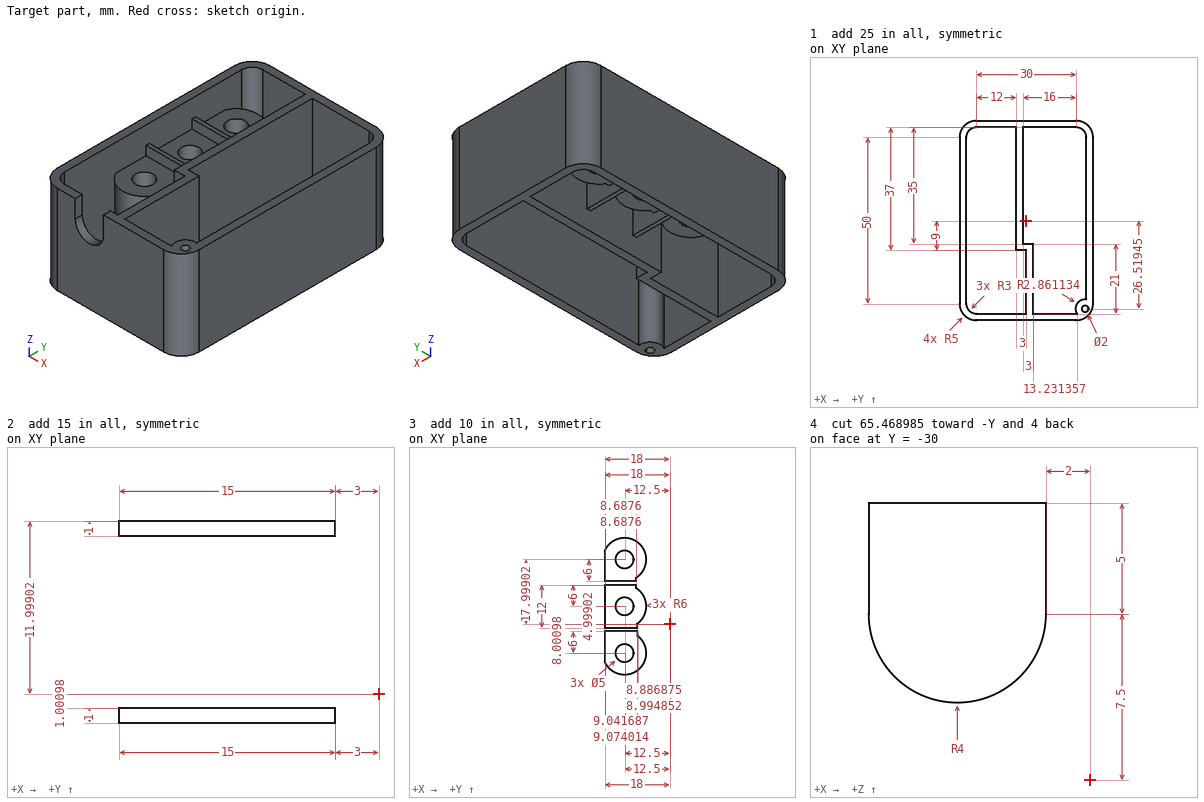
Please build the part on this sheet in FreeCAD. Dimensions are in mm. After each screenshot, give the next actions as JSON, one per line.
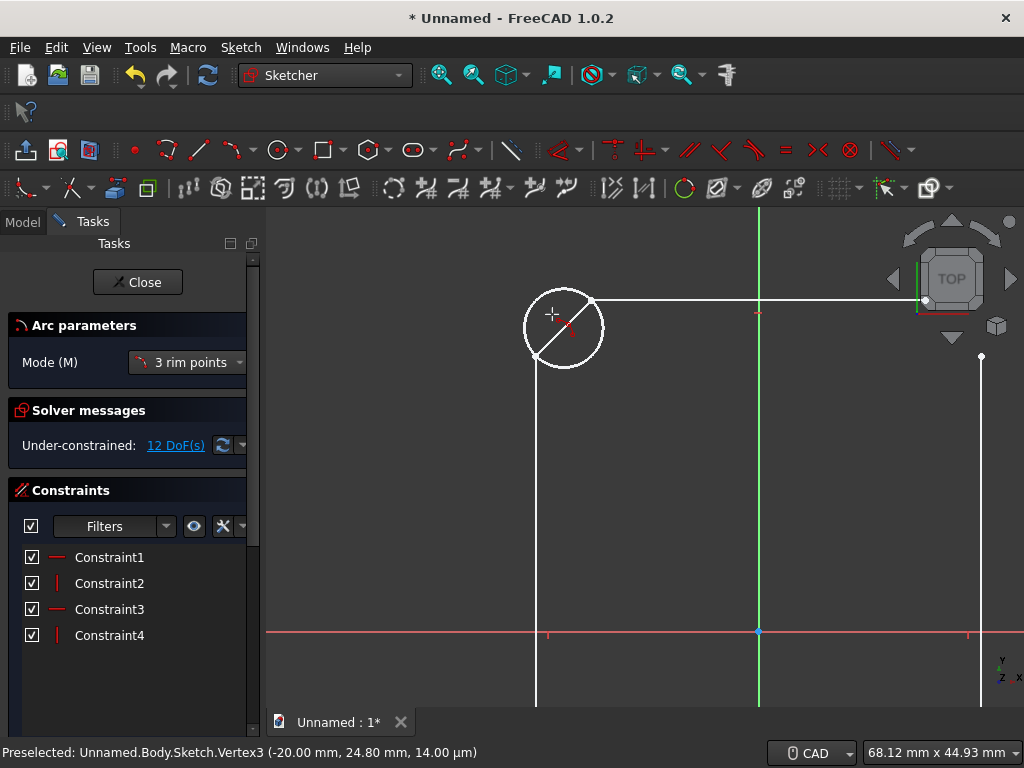
{"action": "left_click", "coordinate": [552, 314]}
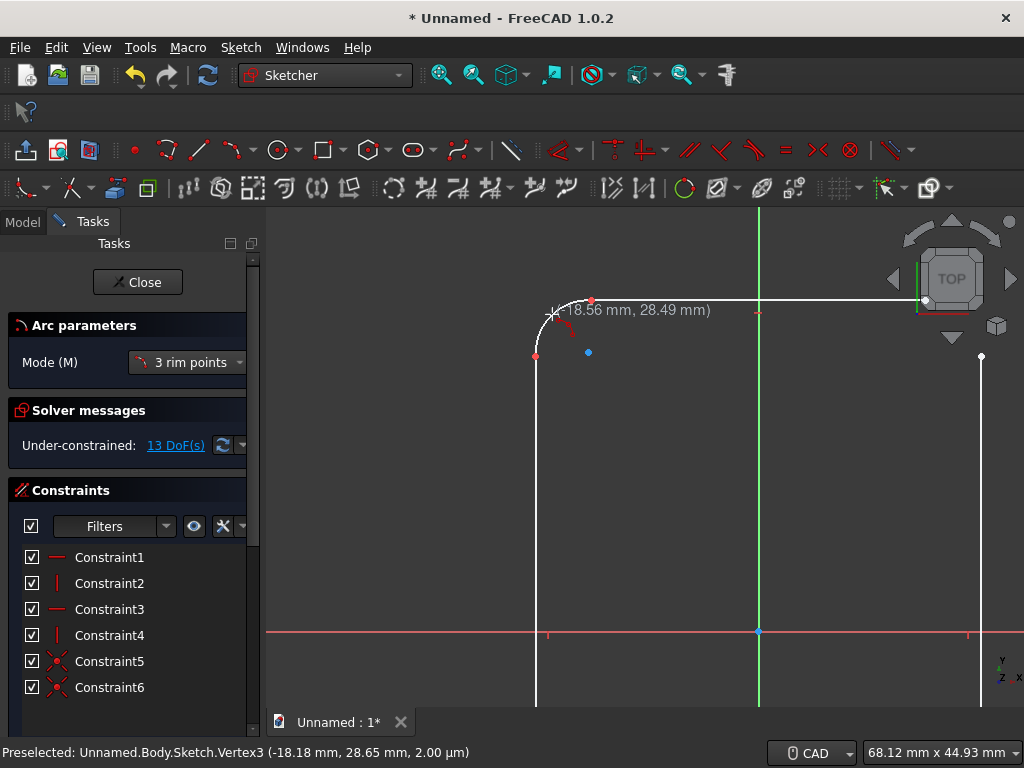
{"action": "scroll", "coordinate": [428, 314], "scroll_direction": "down", "scroll_amount": 4}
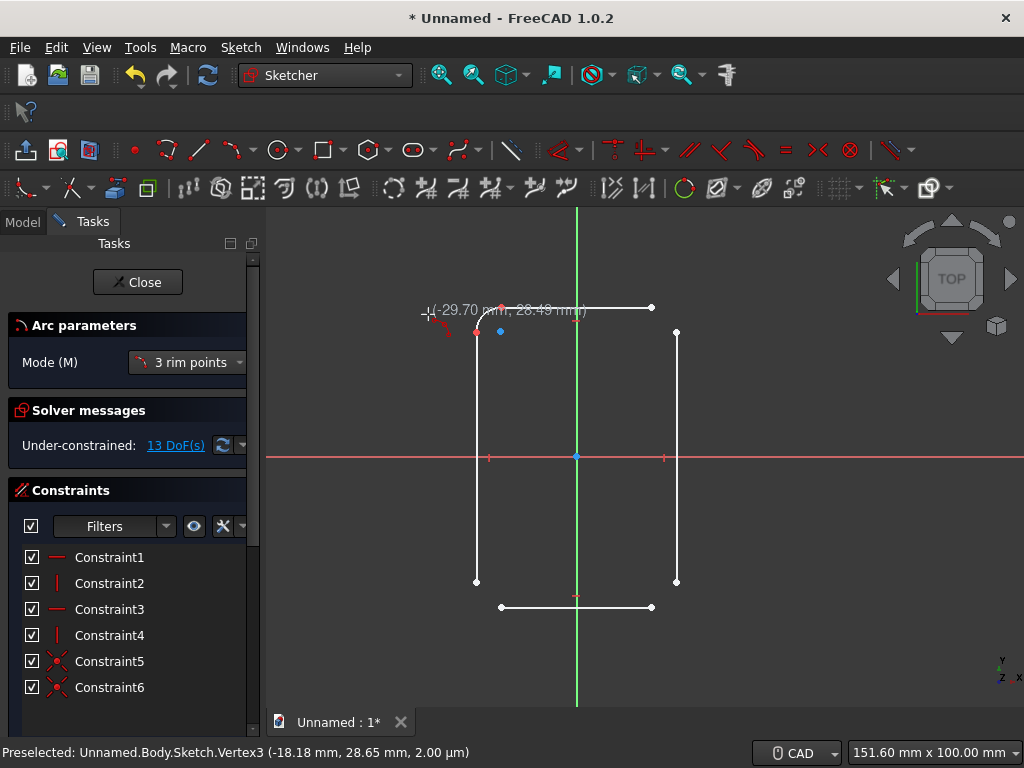
{"action": "left_click", "coordinate": [477, 583]}
{"action": "left_click", "coordinate": [502, 608]}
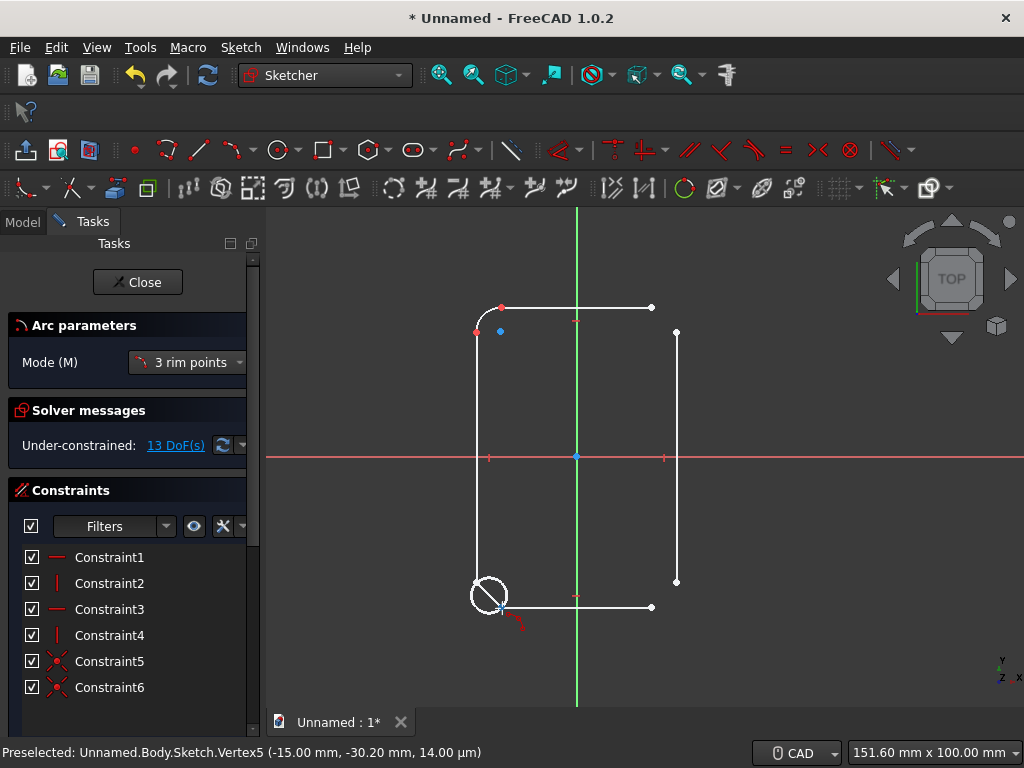
{"action": "scroll", "coordinate": [484, 600], "scroll_direction": "up", "scroll_amount": 4}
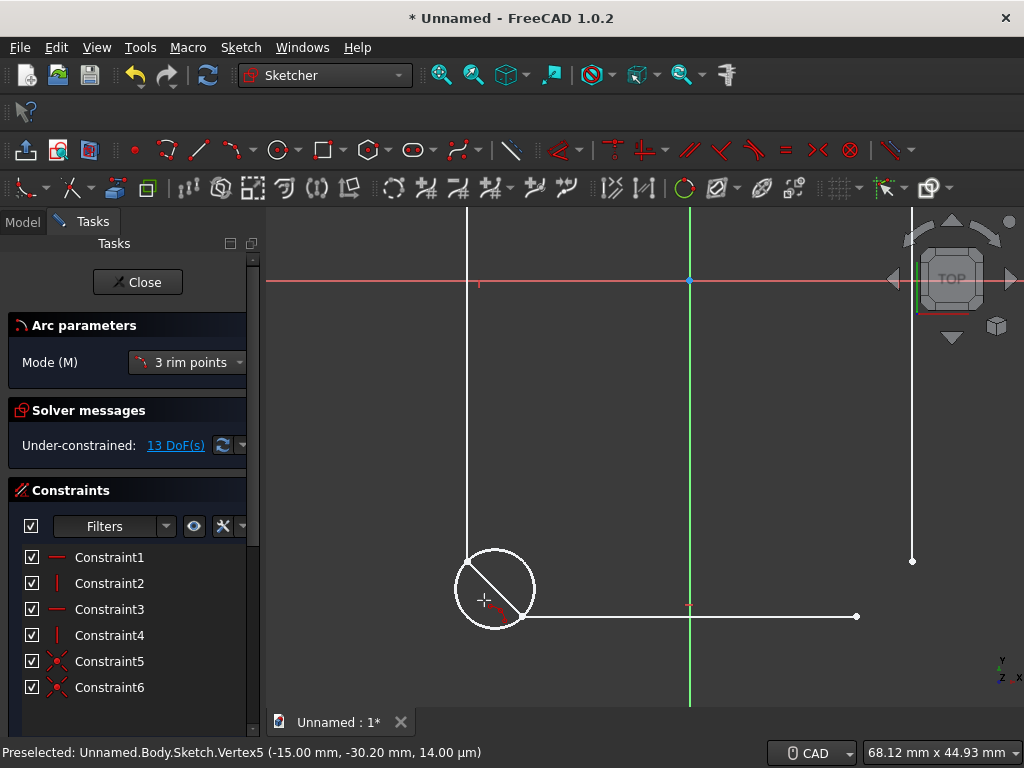
{"action": "left_click", "coordinate": [484, 598]}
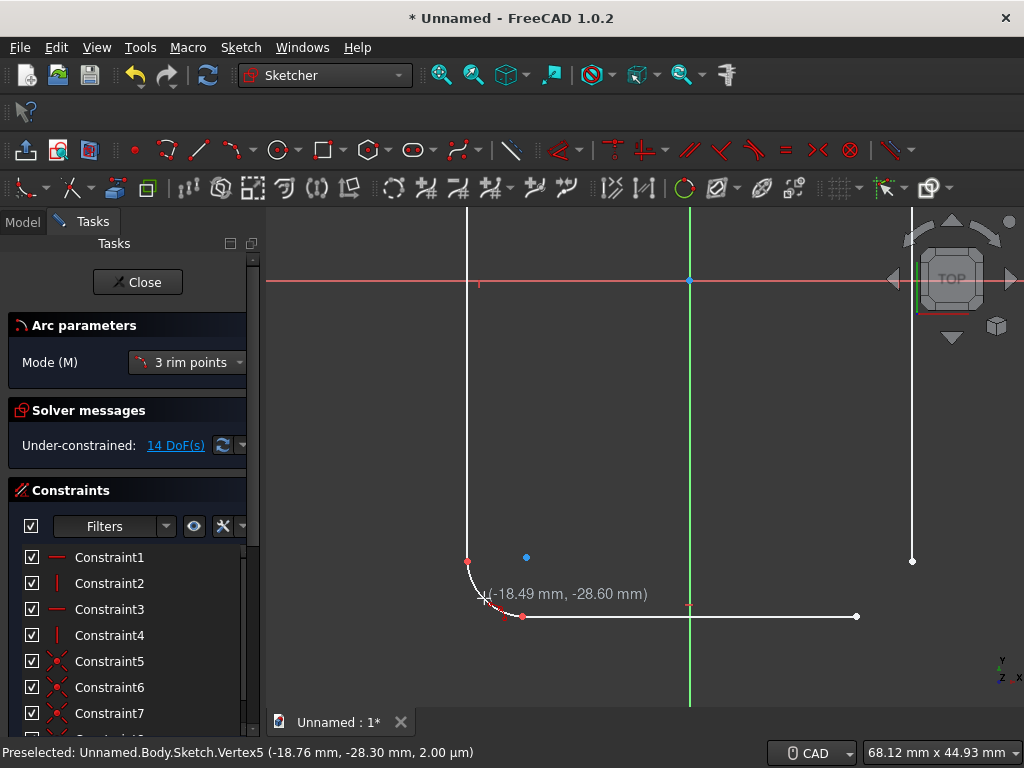
{"action": "left_click", "coordinate": [857, 617]}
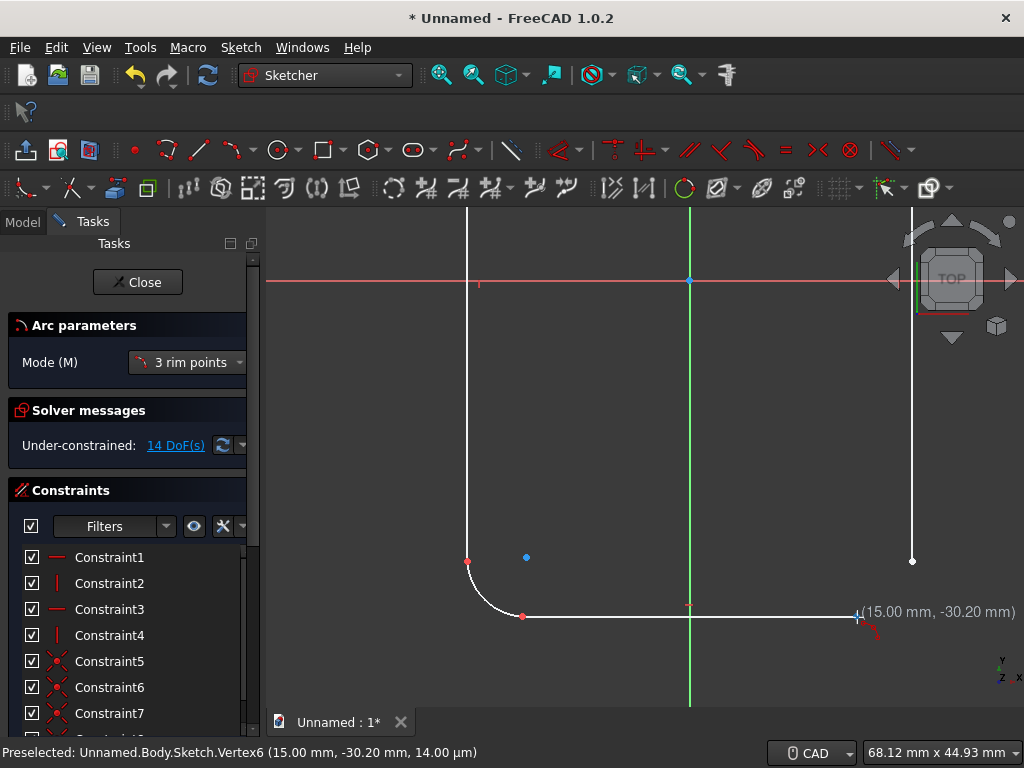
{"action": "scroll", "coordinate": [484, 601], "scroll_direction": "down", "scroll_amount": 4}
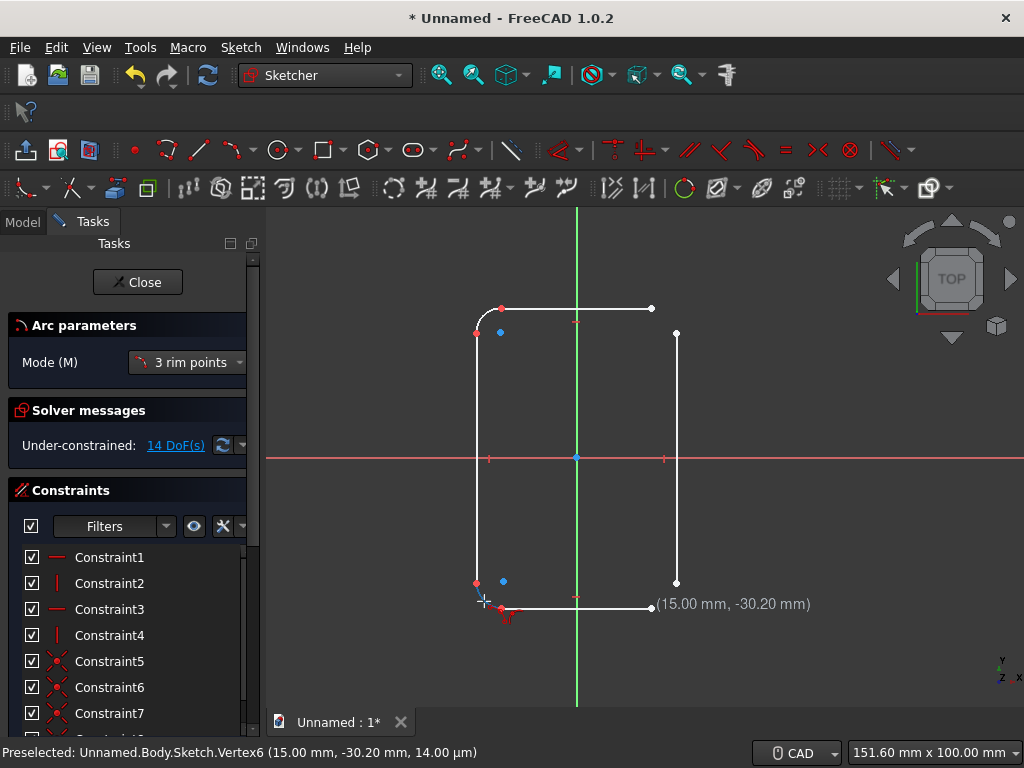
{"action": "left_click", "coordinate": [677, 584]}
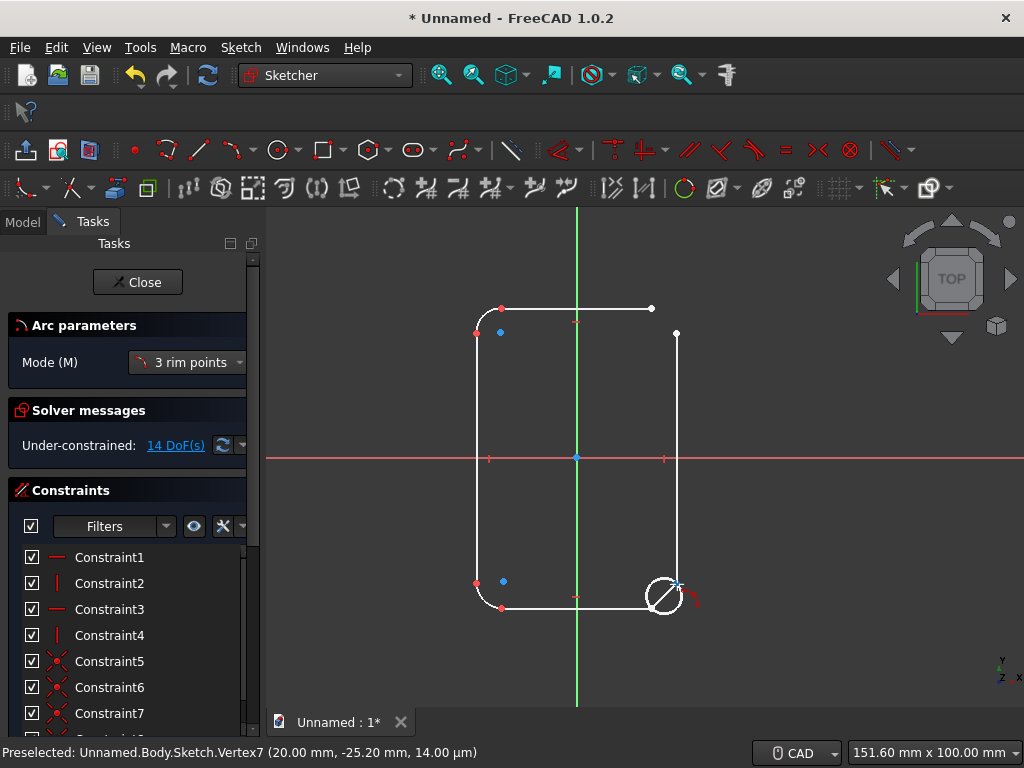
{"action": "scroll", "coordinate": [669, 600], "scroll_direction": "up", "scroll_amount": 4}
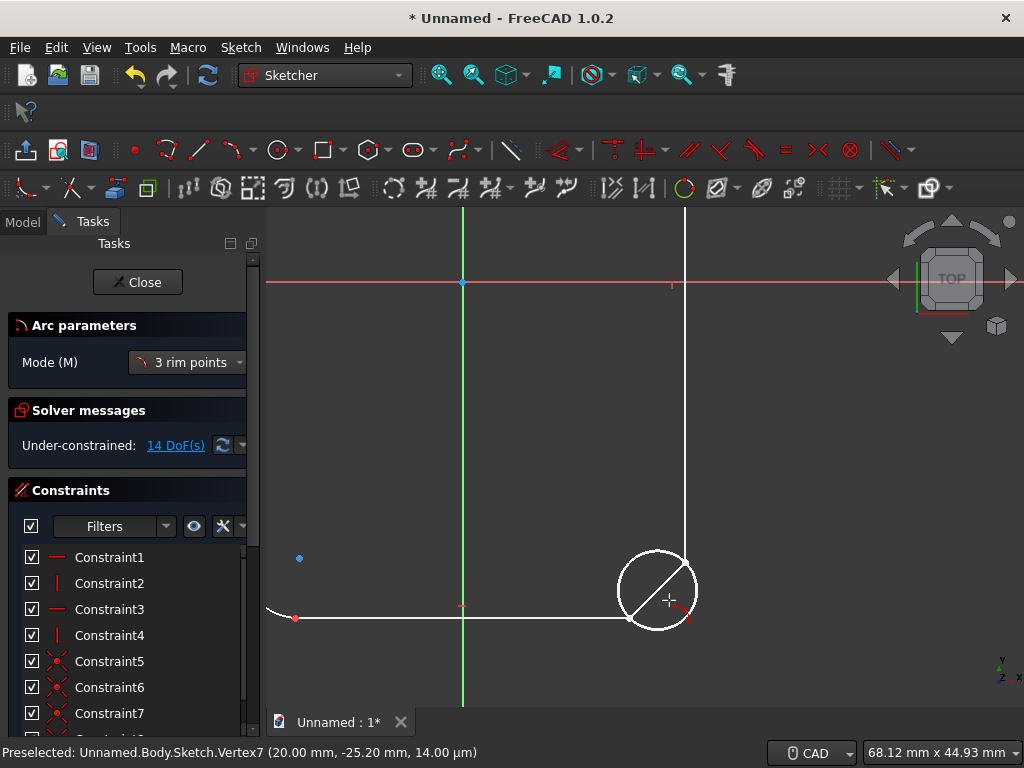
{"action": "left_click", "coordinate": [669, 600]}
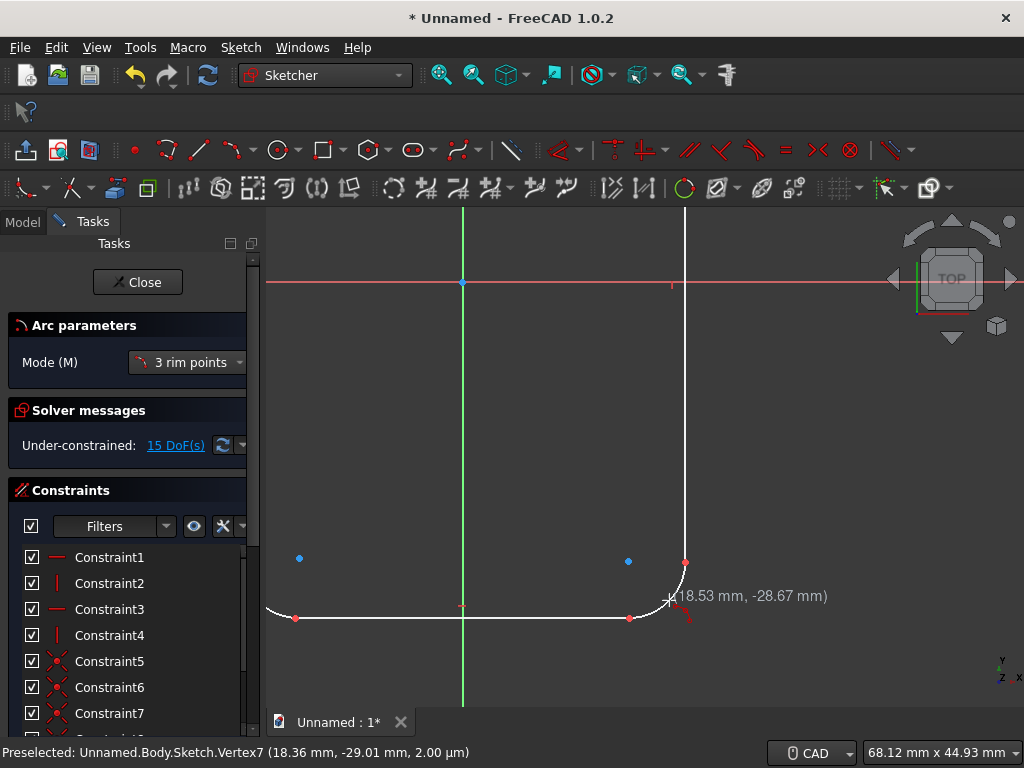
{"action": "scroll", "coordinate": [669, 600], "scroll_direction": "down", "scroll_amount": 4}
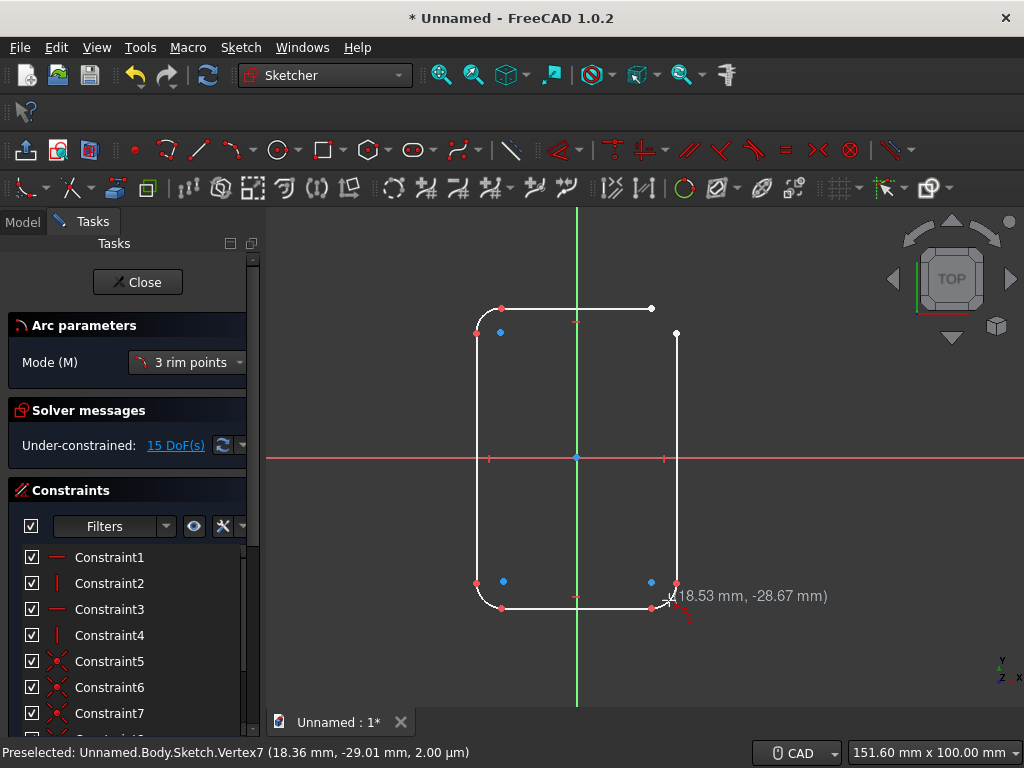
{"action": "left_click", "coordinate": [677, 334]}
{"action": "left_click", "coordinate": [652, 309]}